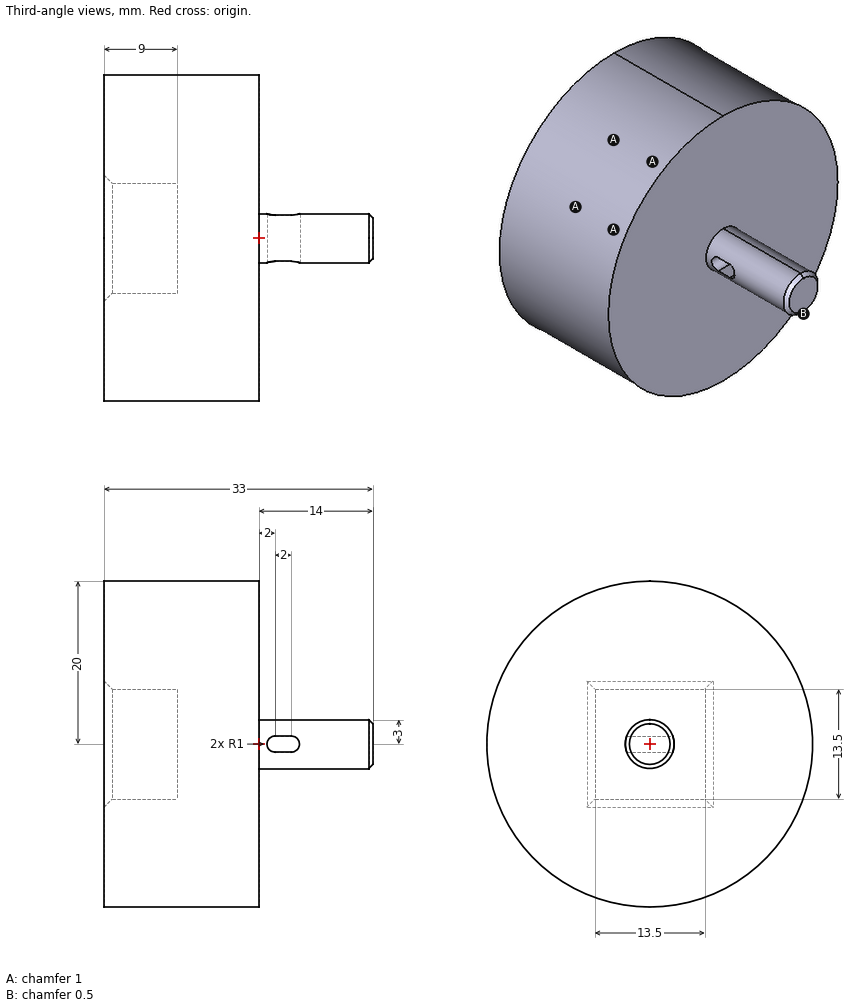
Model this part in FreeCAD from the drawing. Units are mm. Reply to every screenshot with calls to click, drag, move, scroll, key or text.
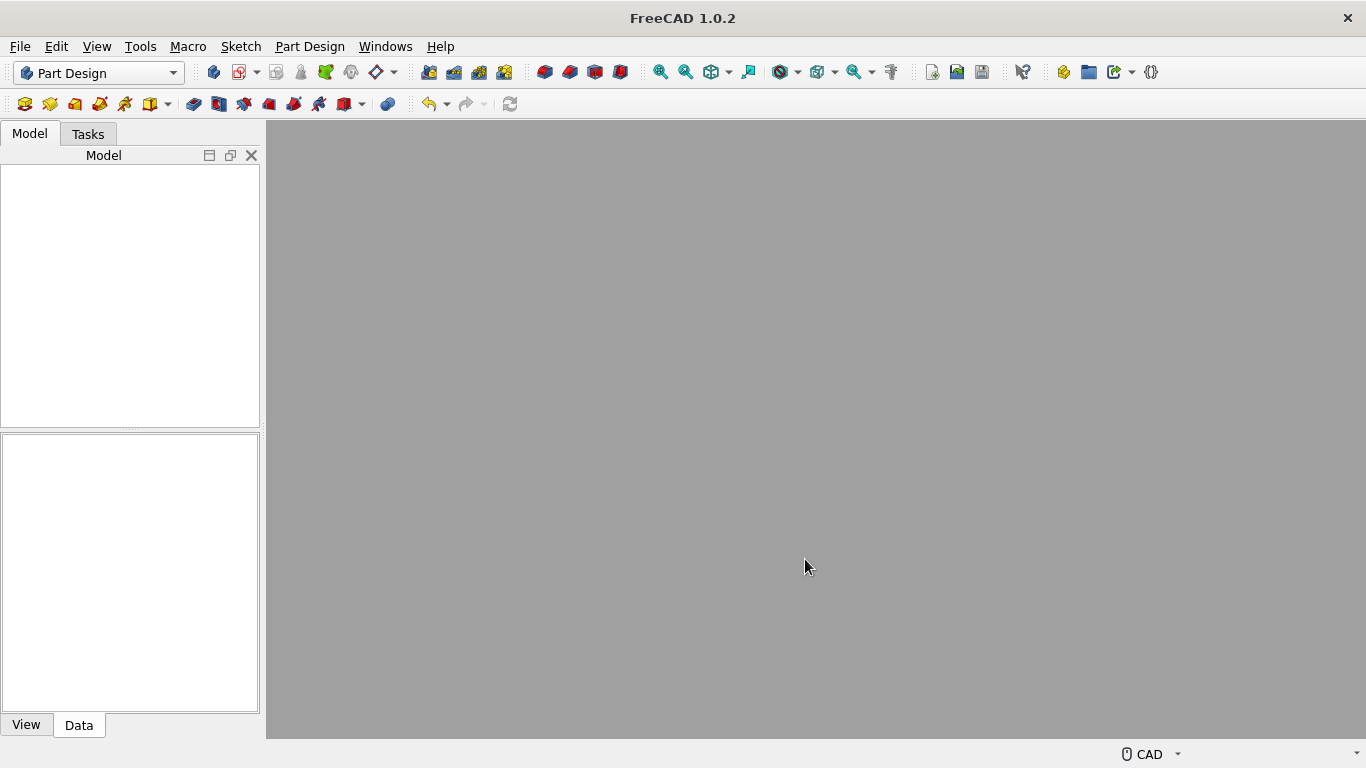
click(932, 72)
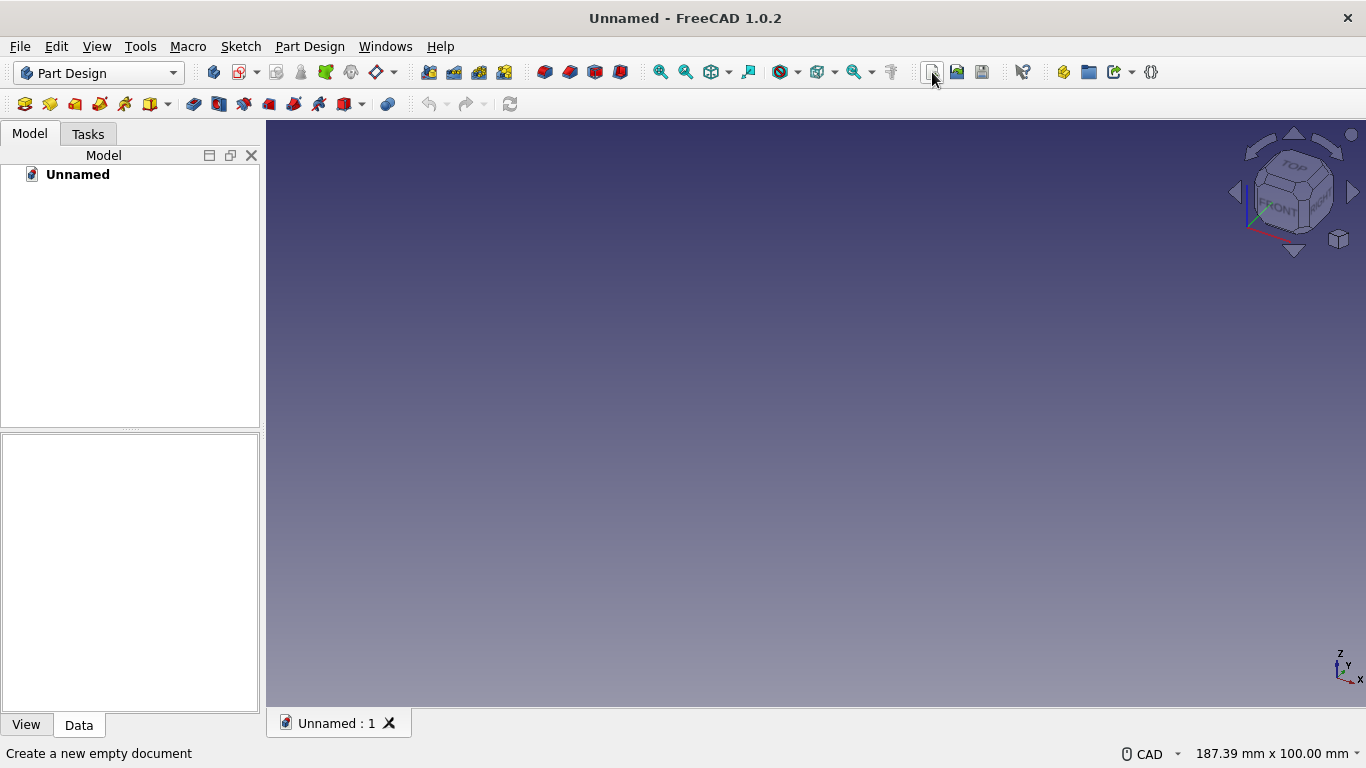
click(238, 72)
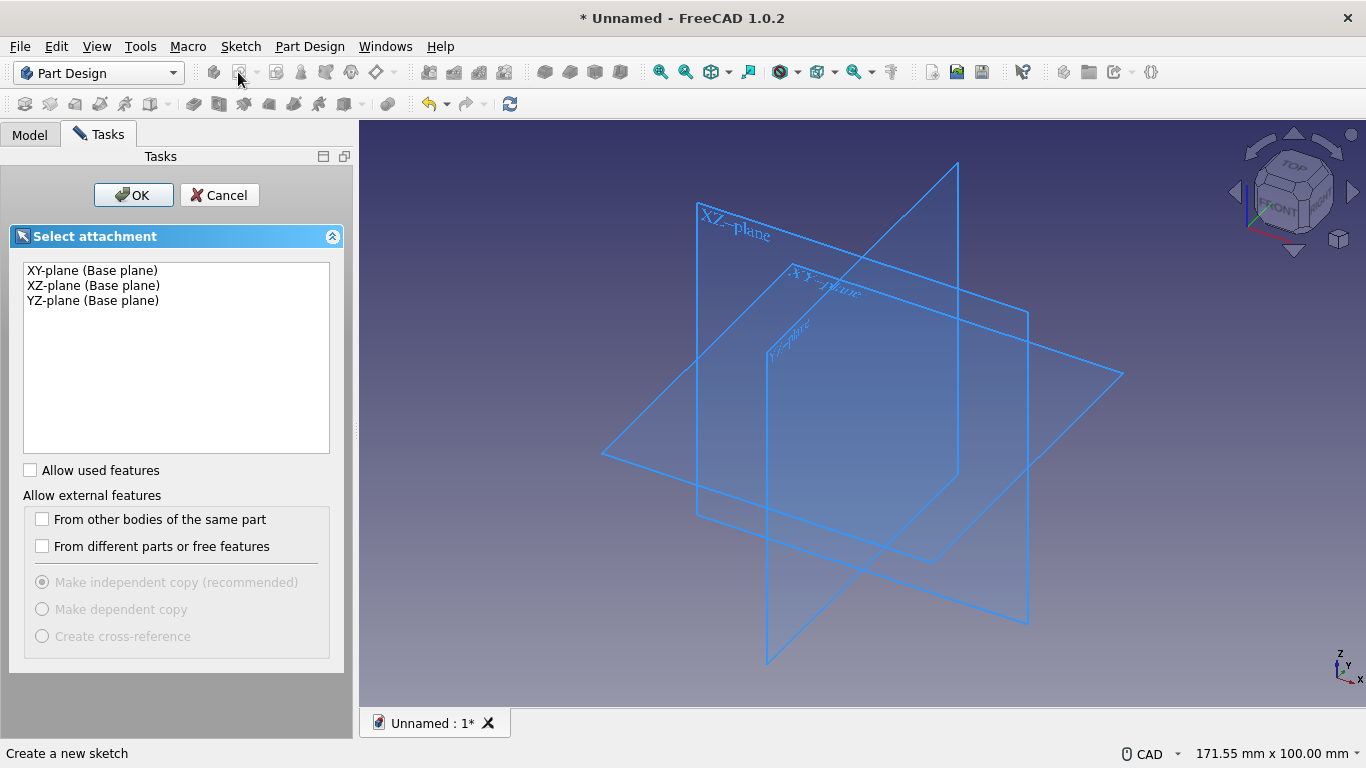
click(84, 286)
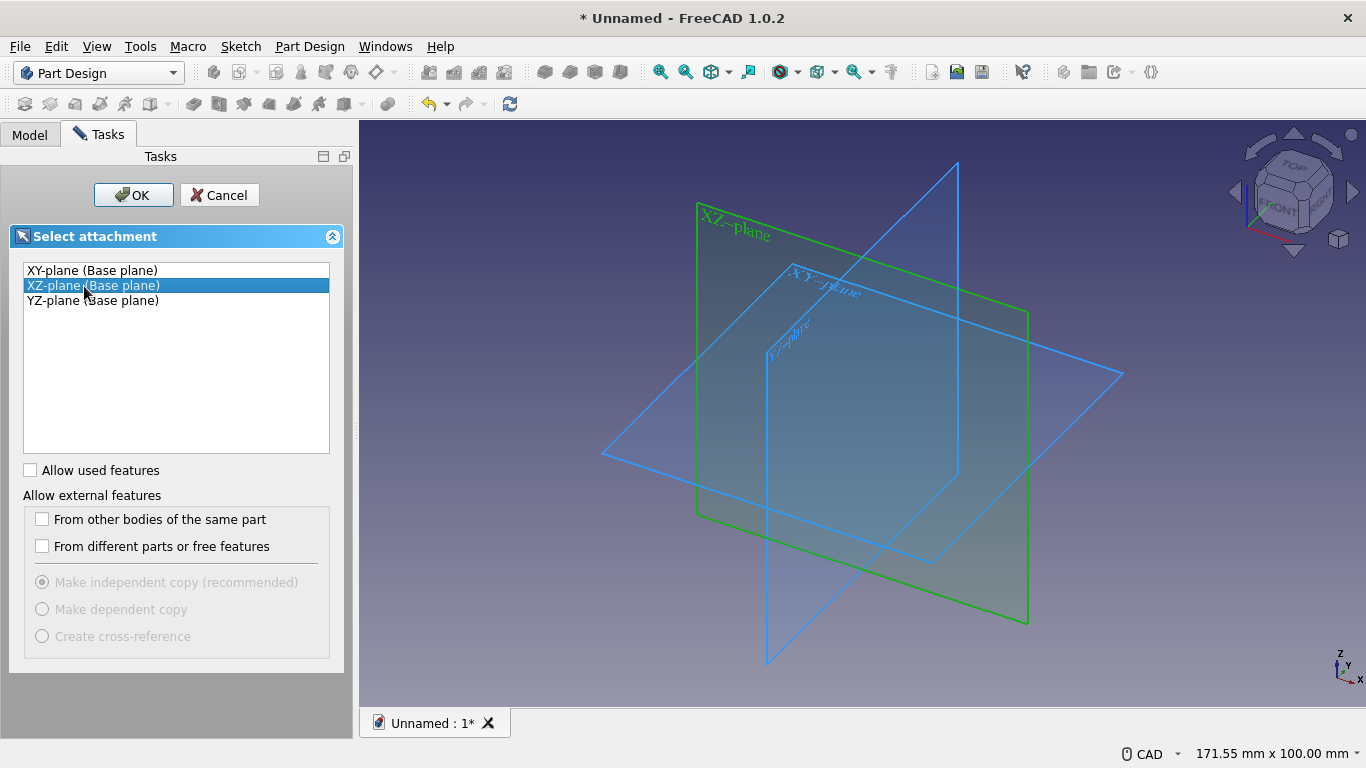
click(134, 195)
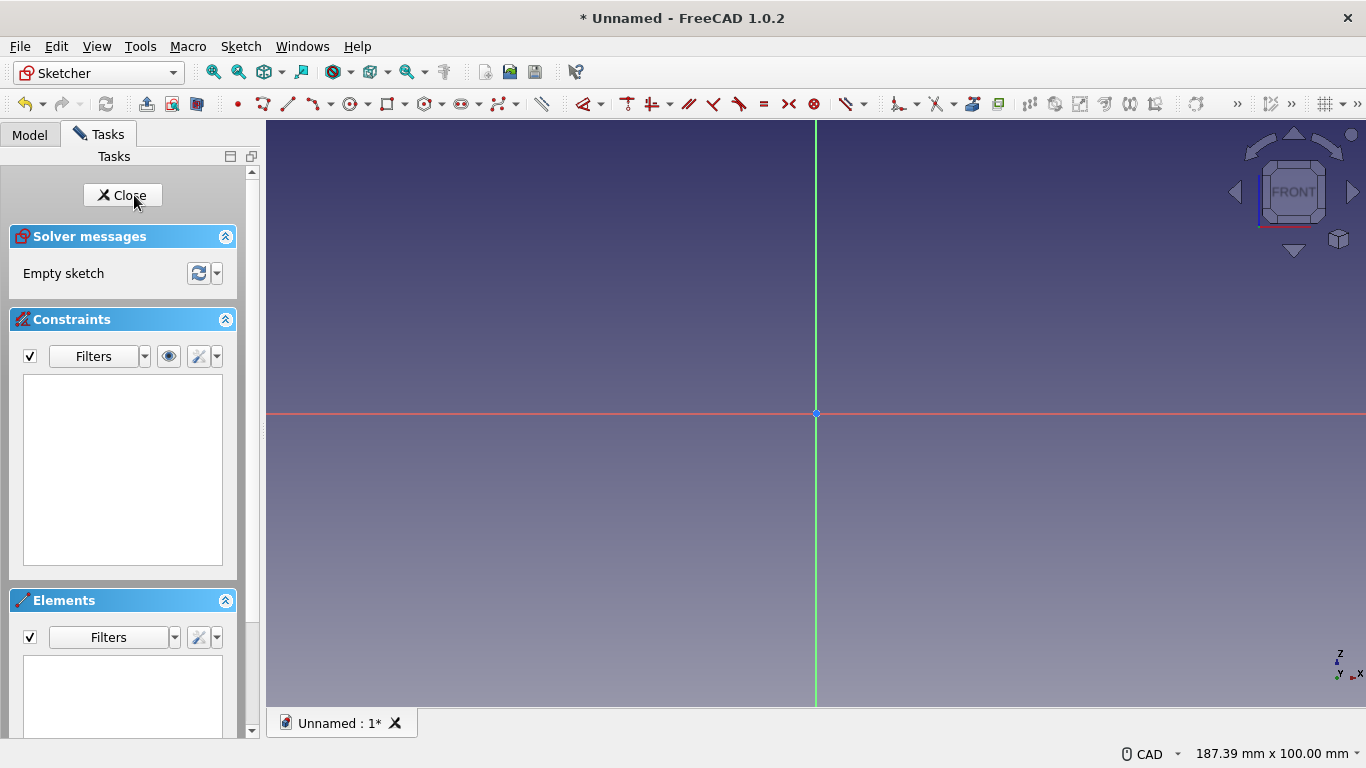
scroll(825, 329, up, 6)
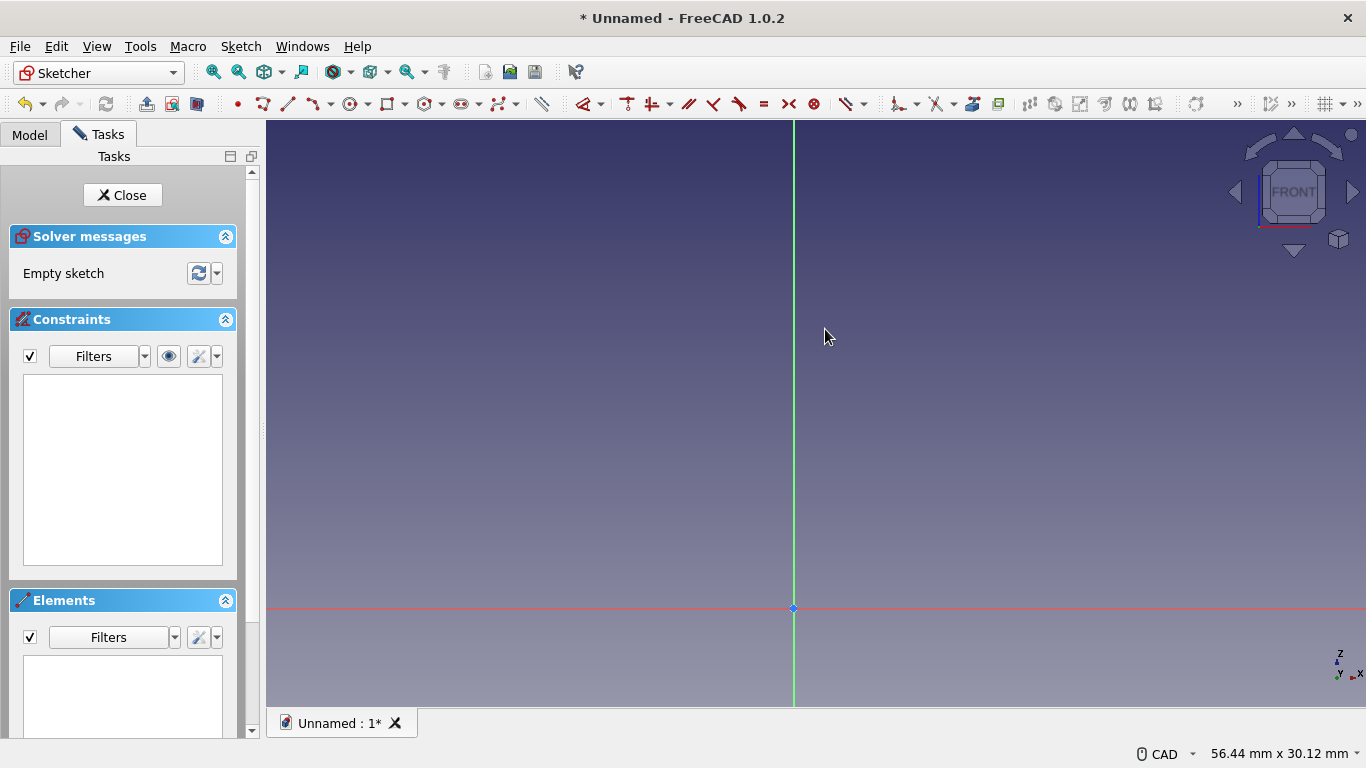
click(263, 104)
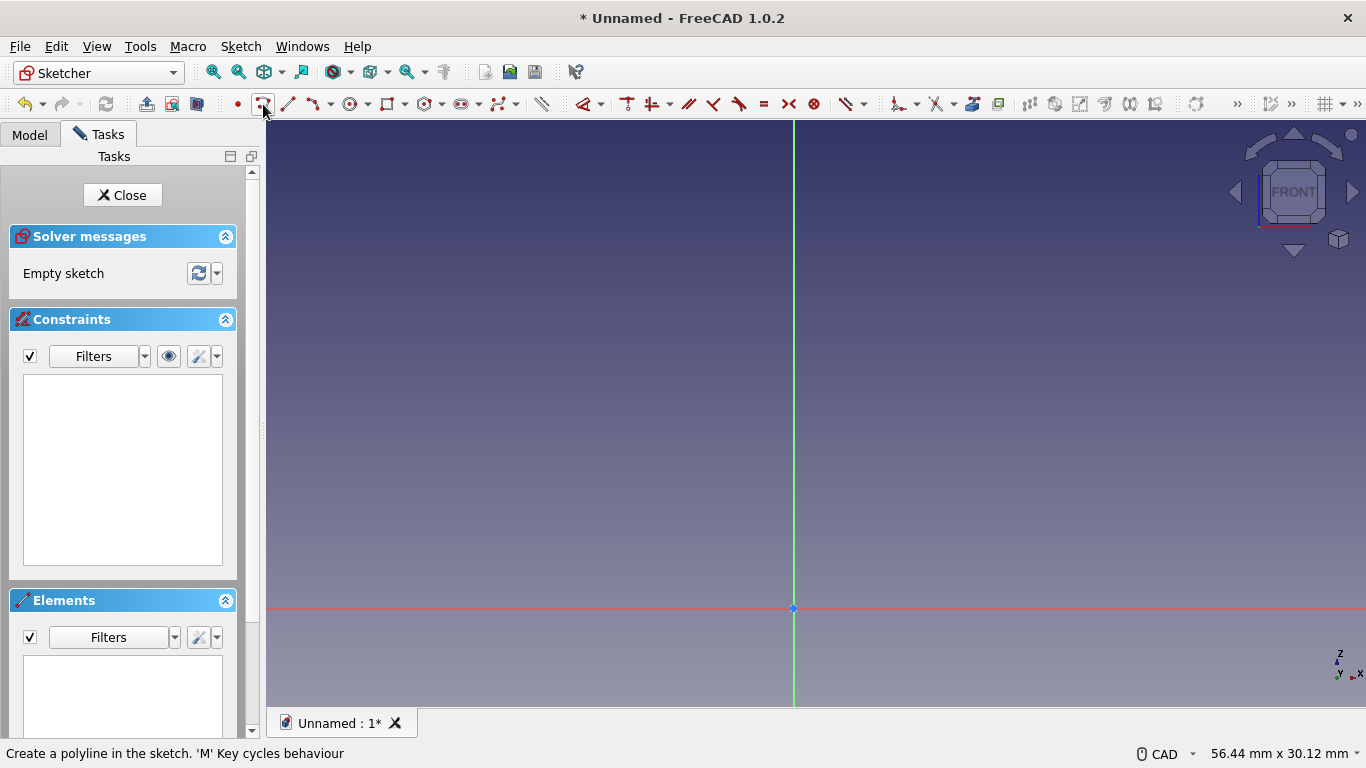
click(794, 550)
click(1067, 550)
click(1067, 609)
click(424, 600)
click(424, 219)
click(785, 219)
click(794, 551)
key(Escape)
key(Escape)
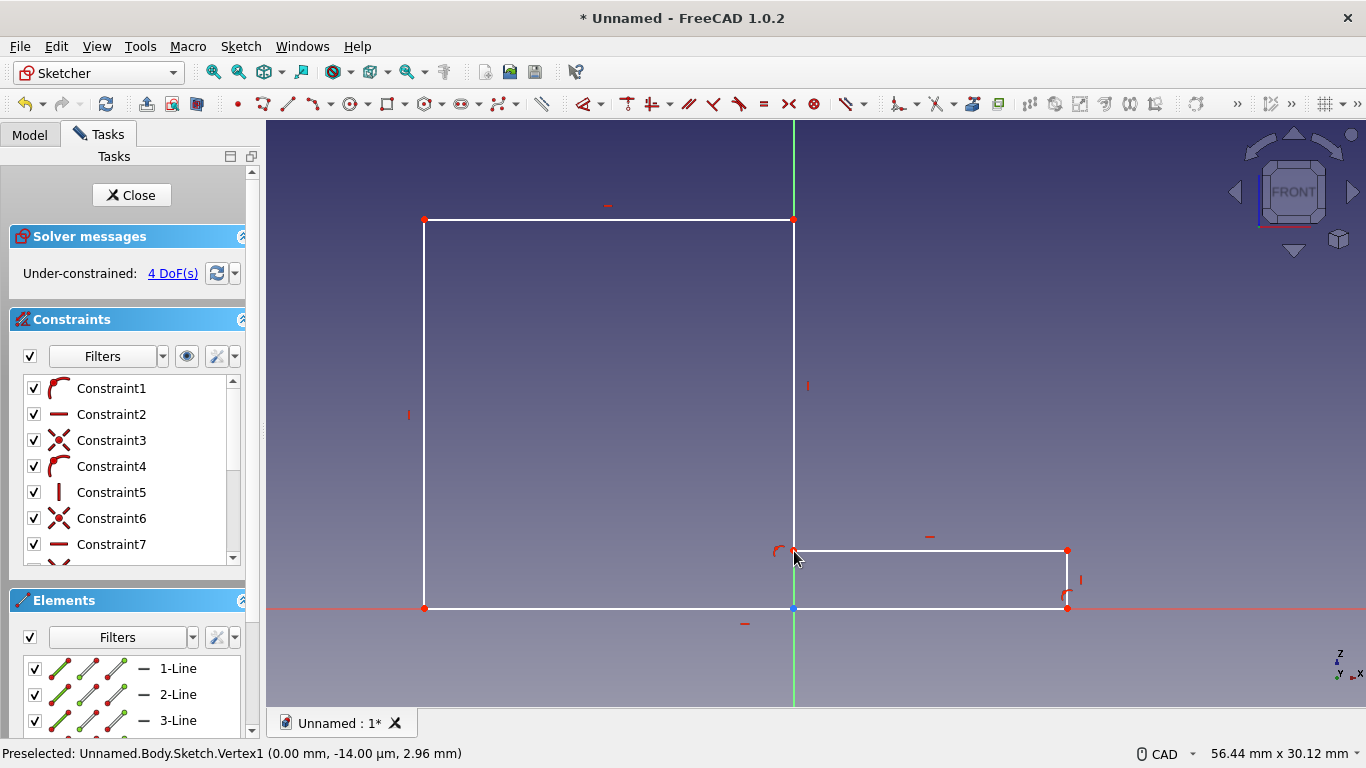
click(1067, 568)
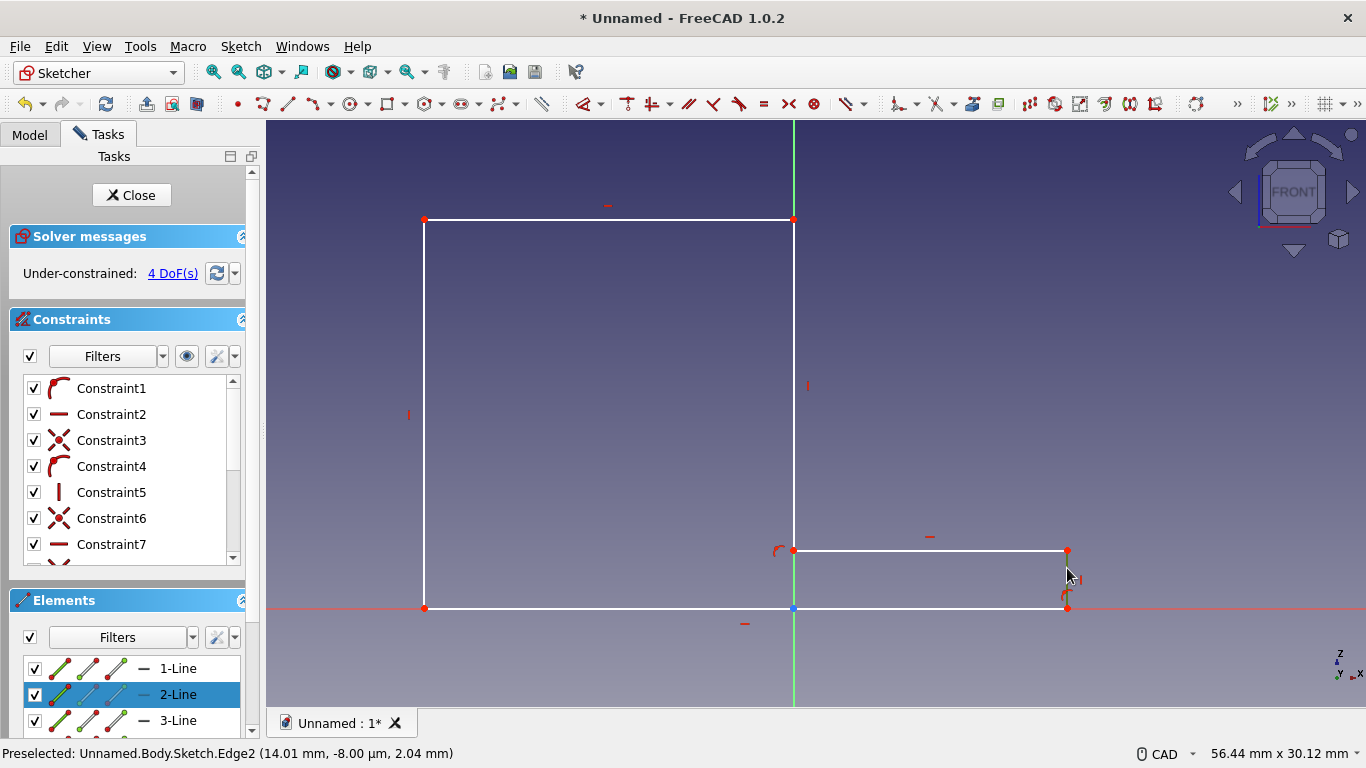
key(i)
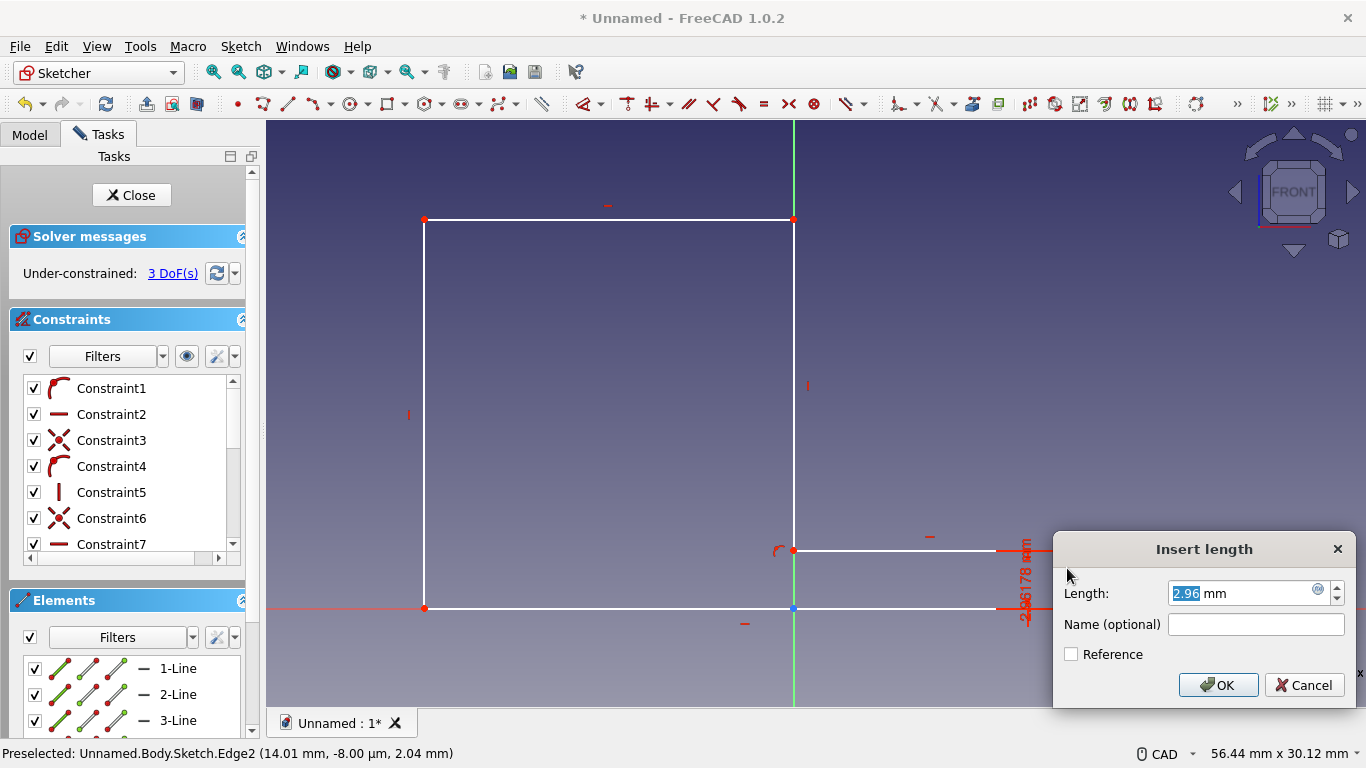
text(3)
key(Return)